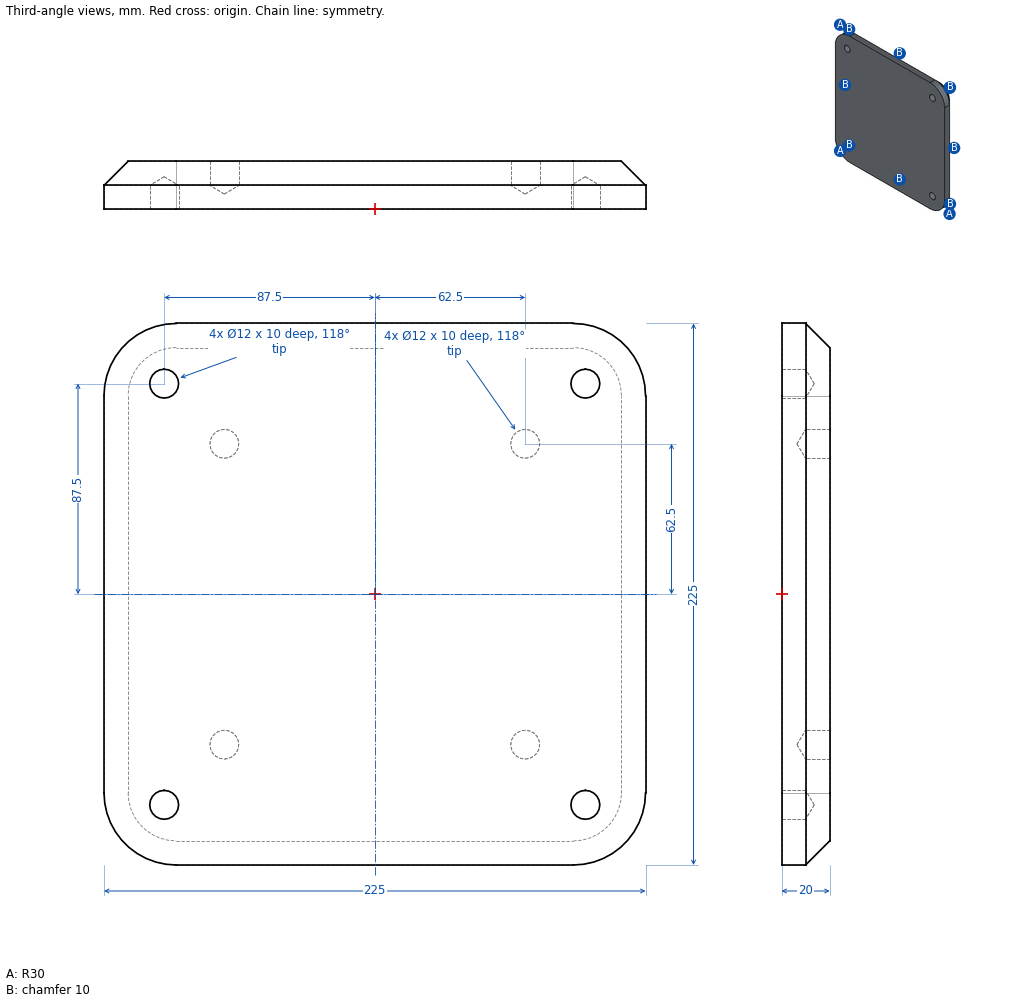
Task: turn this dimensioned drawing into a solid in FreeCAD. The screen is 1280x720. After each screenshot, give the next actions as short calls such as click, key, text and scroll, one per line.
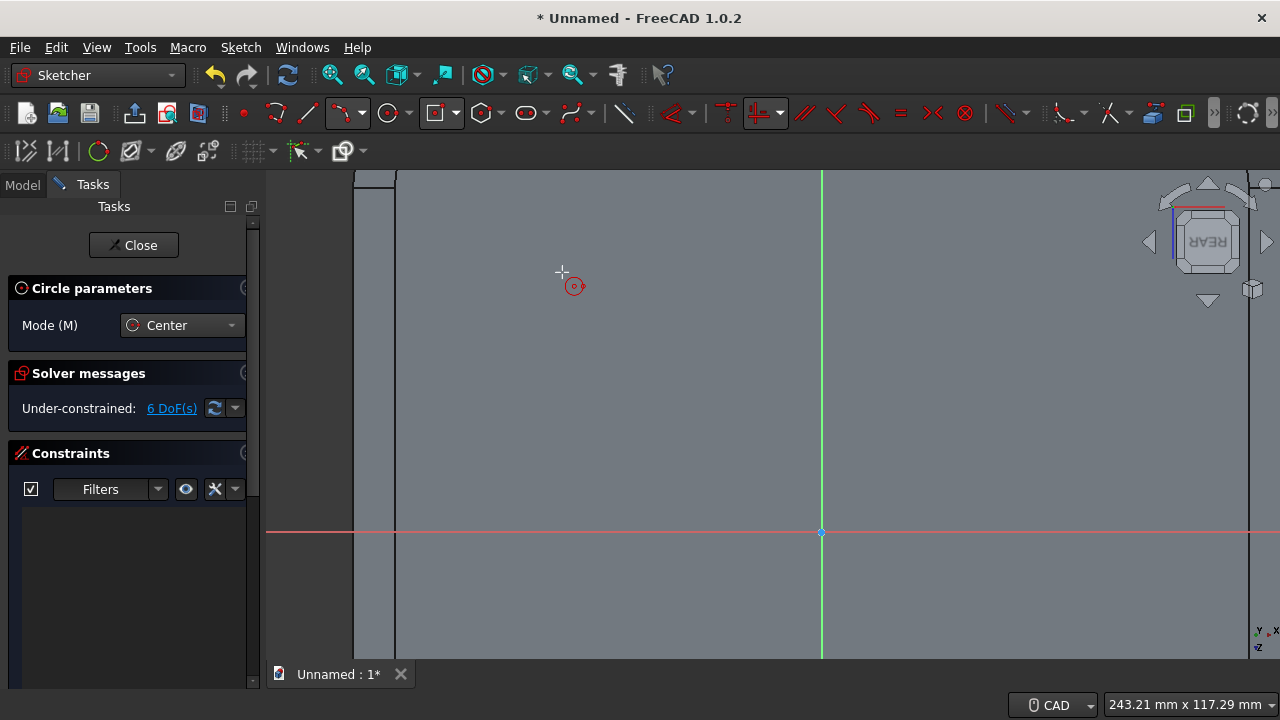
click(561, 272)
click(579, 254)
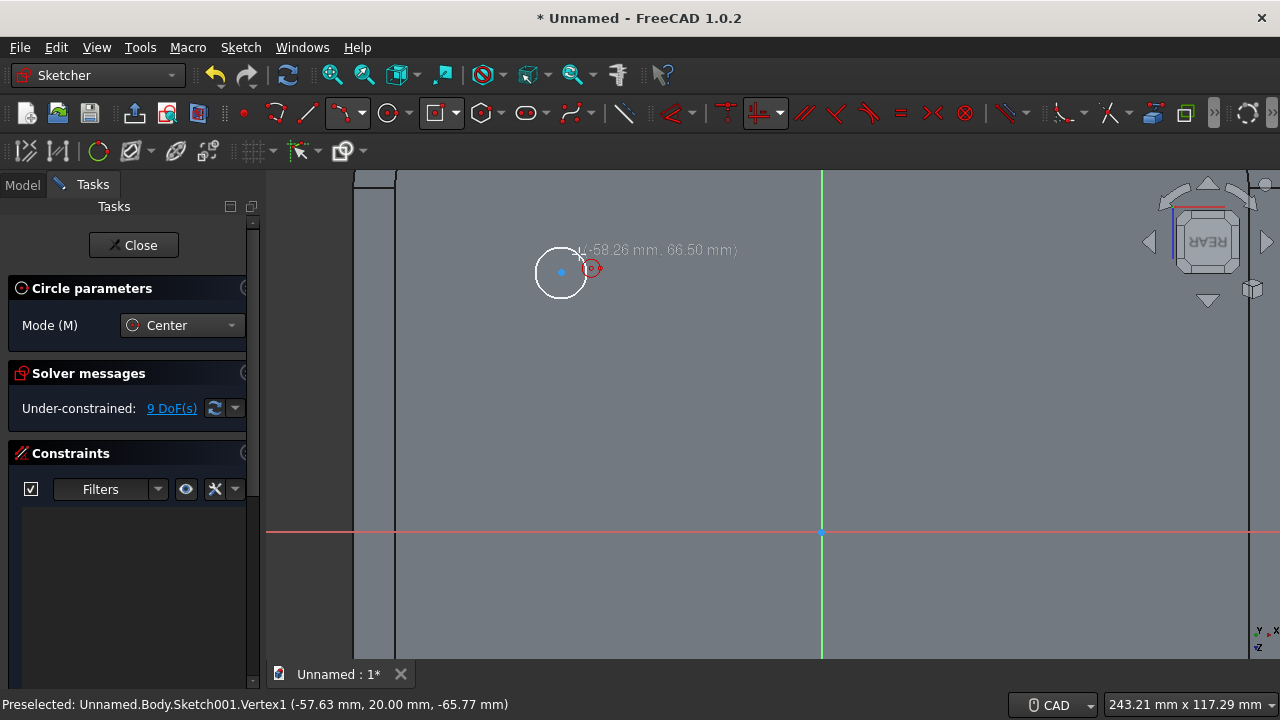
click(1082, 272)
click(1100, 254)
key(Escape)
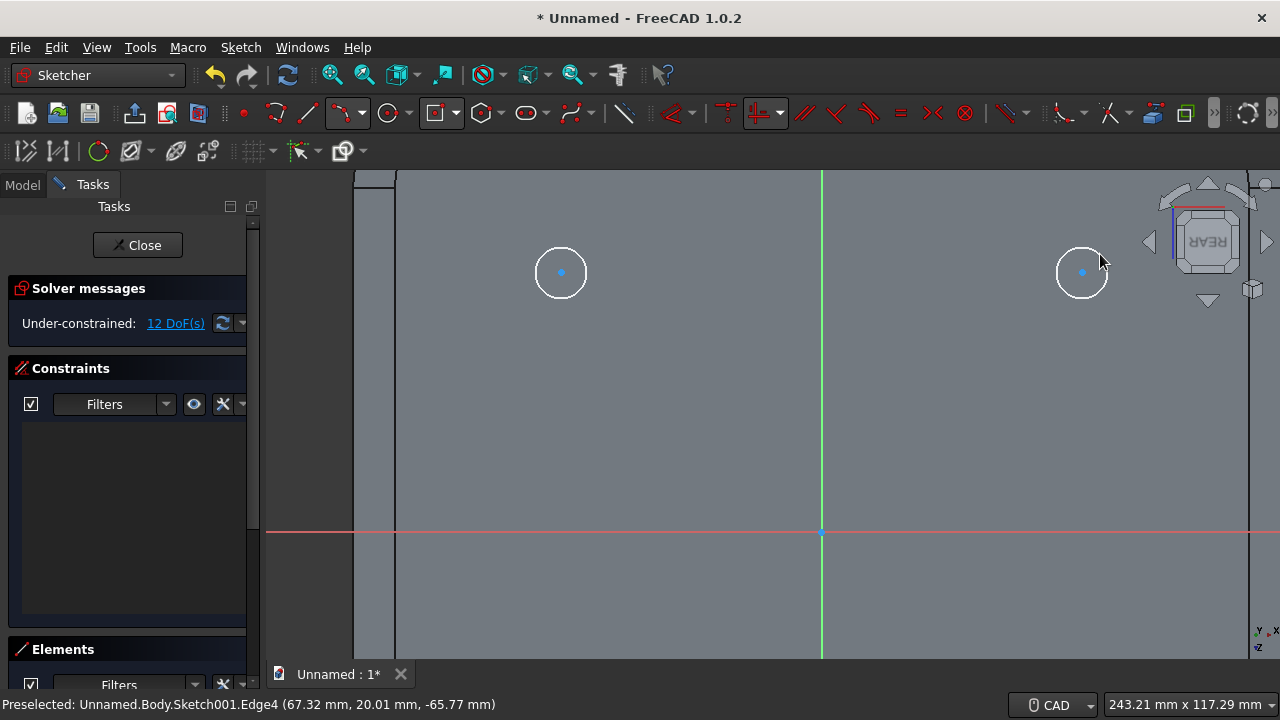
scroll(562, 271, down, 3)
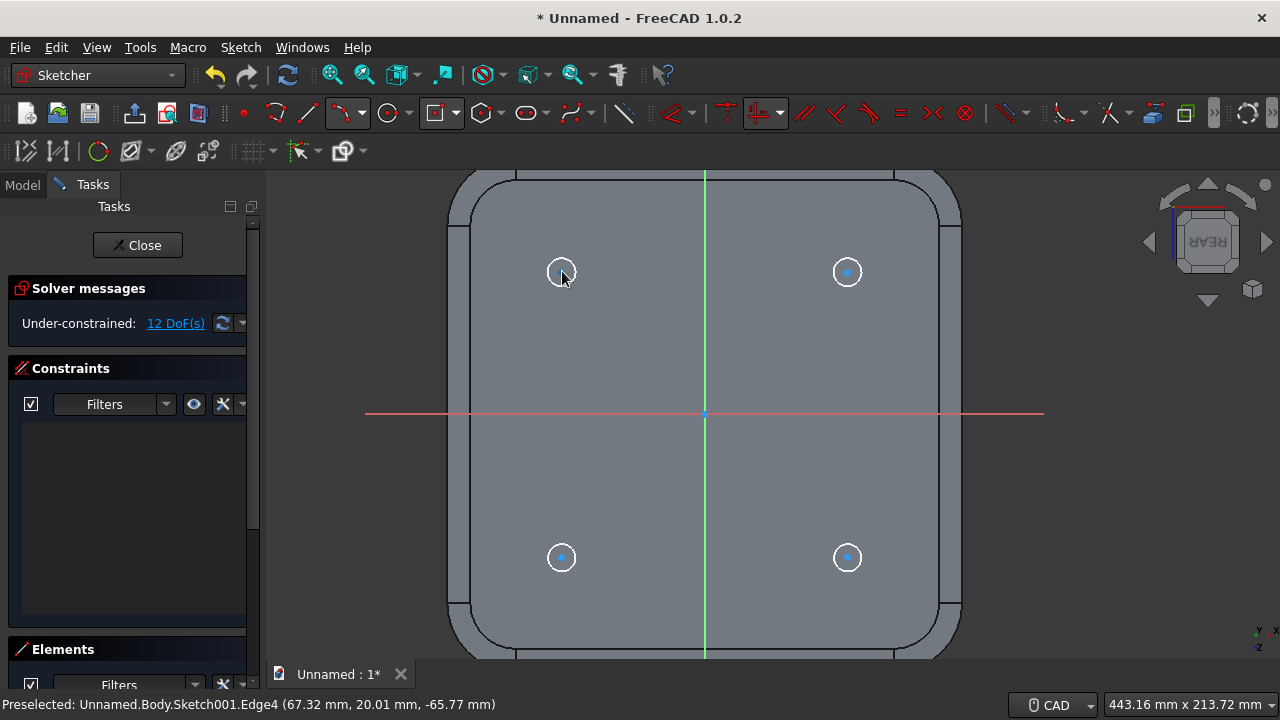
click(857, 548)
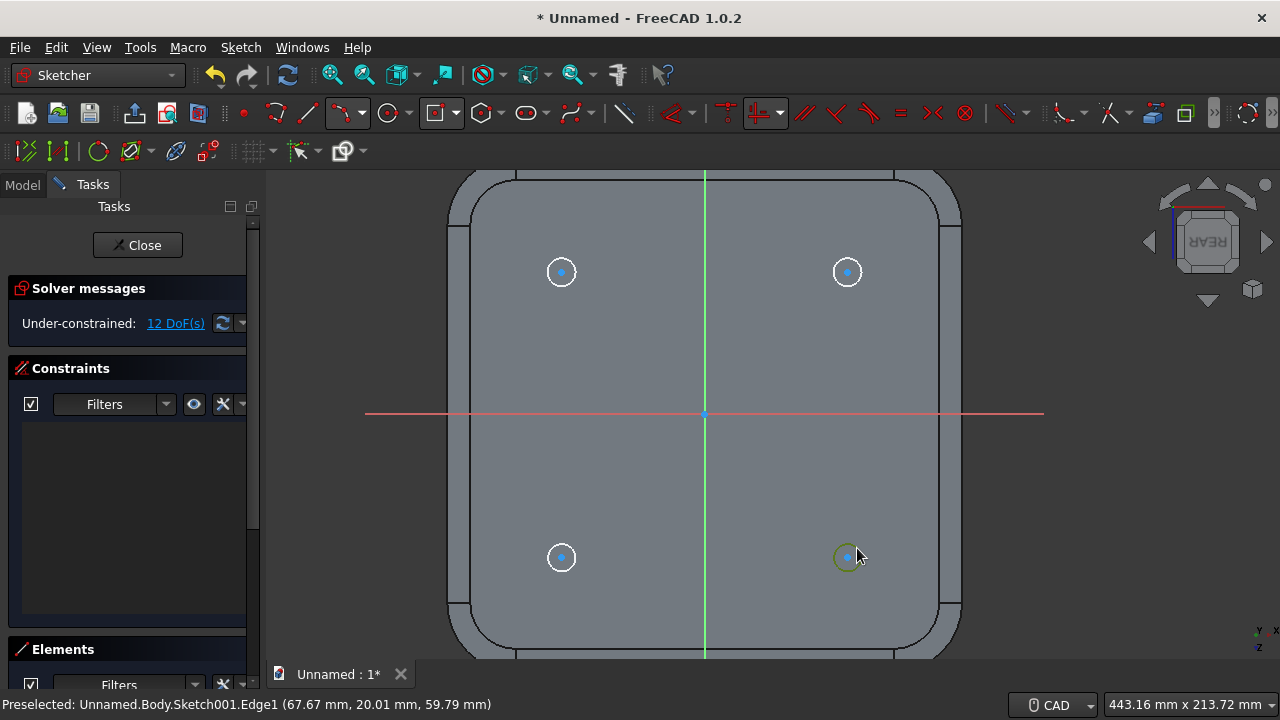
click(571, 548)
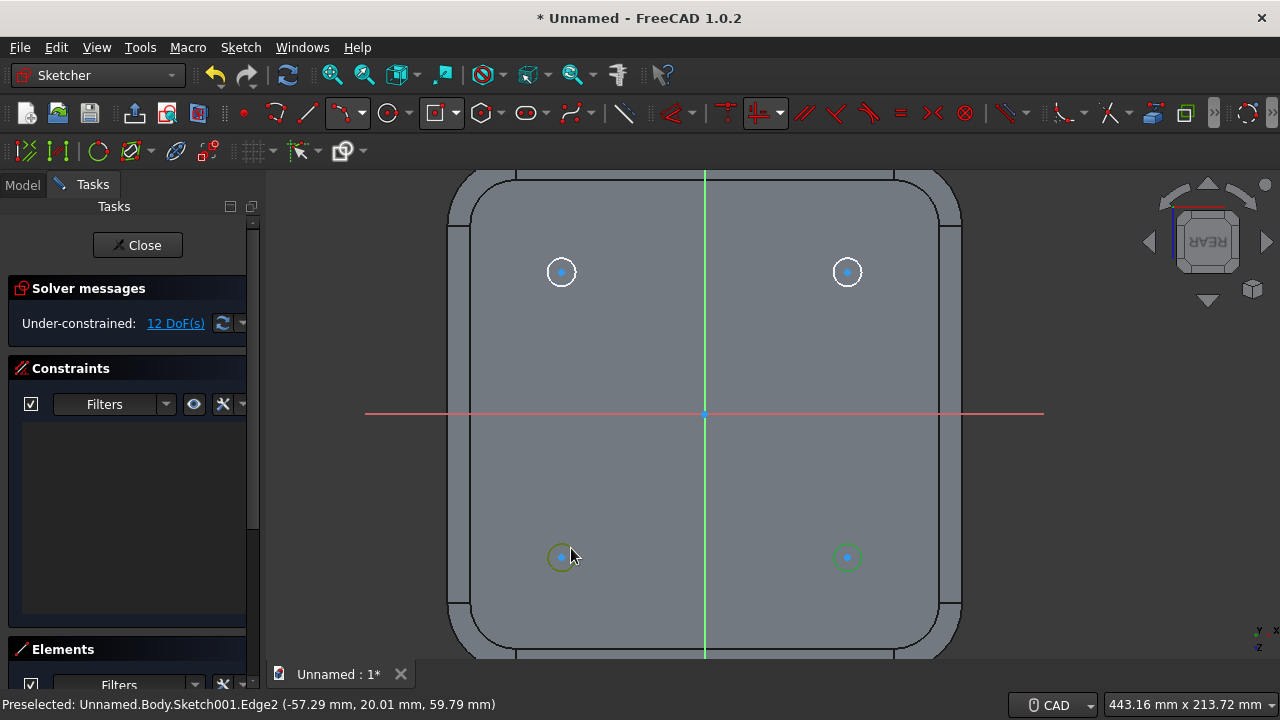
click(571, 262)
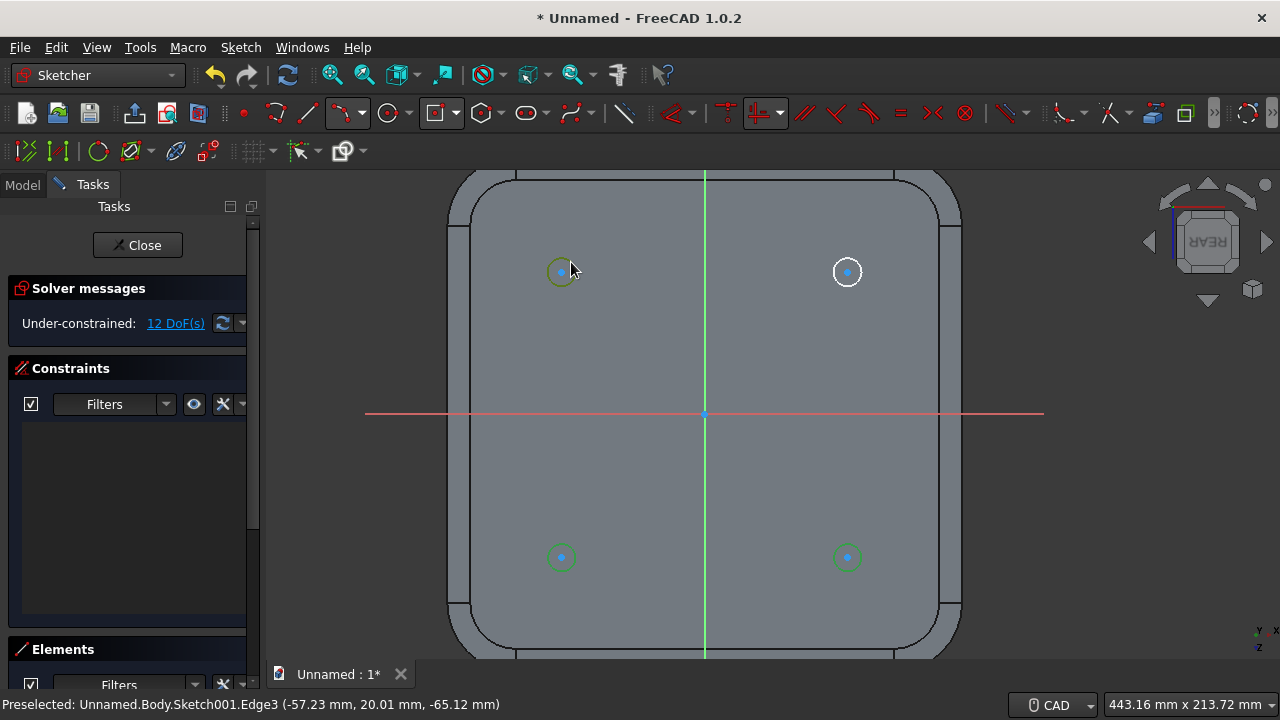
click(857, 262)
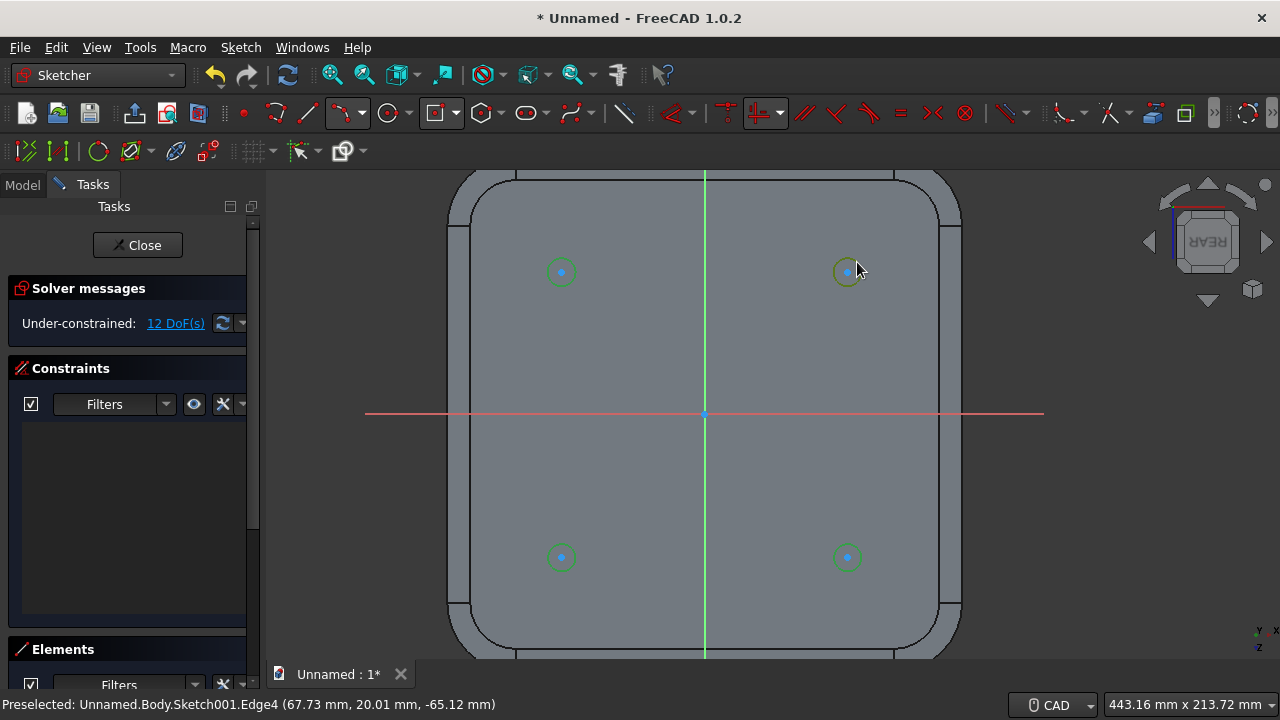
click(902, 114)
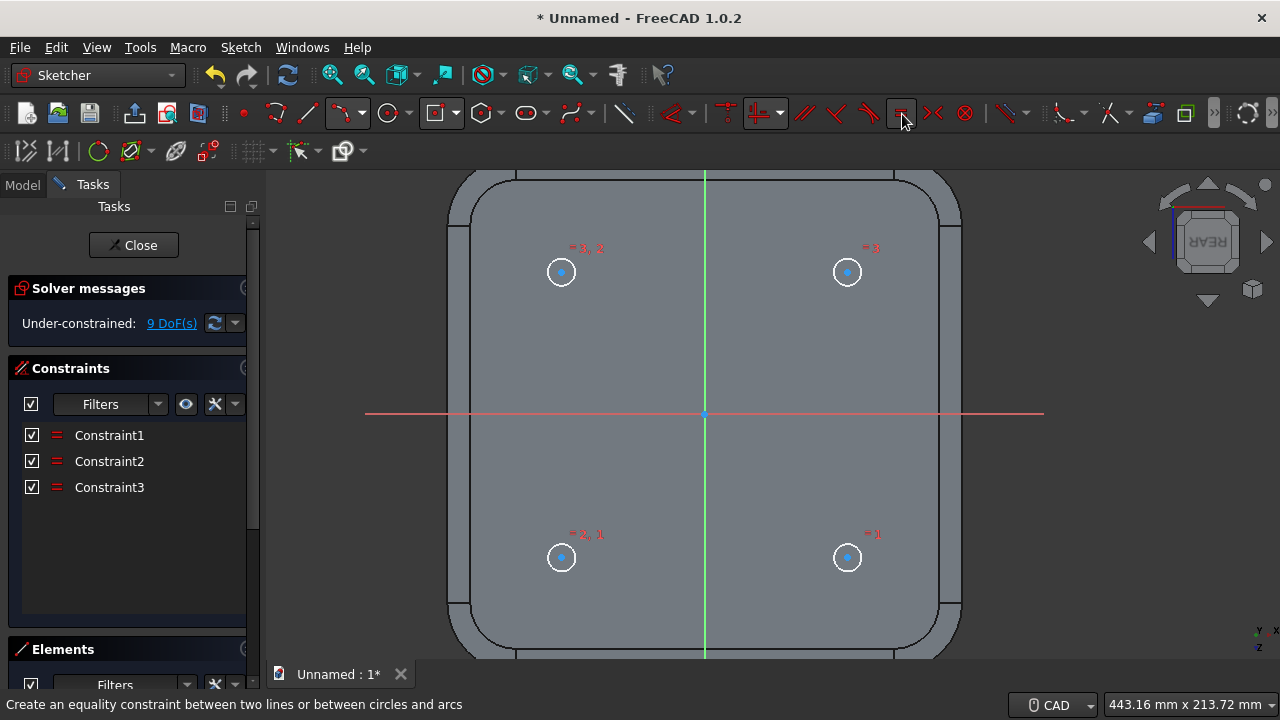
click(848, 558)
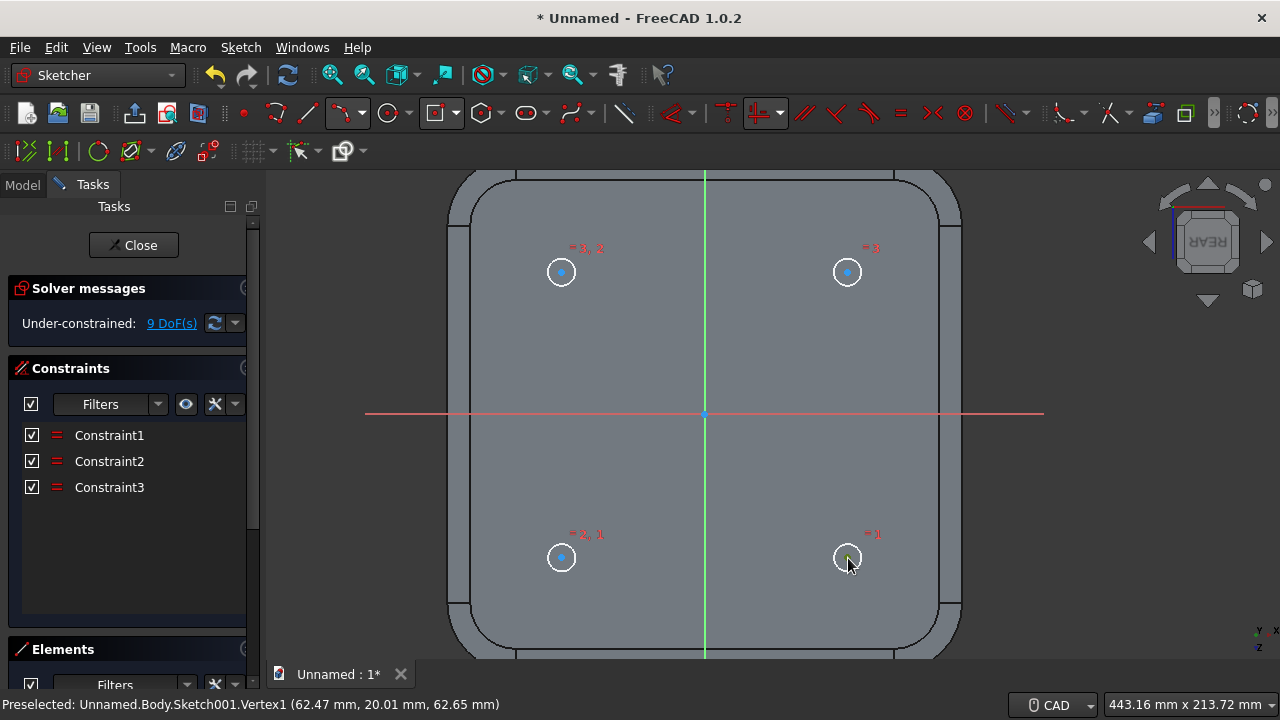
click(562, 558)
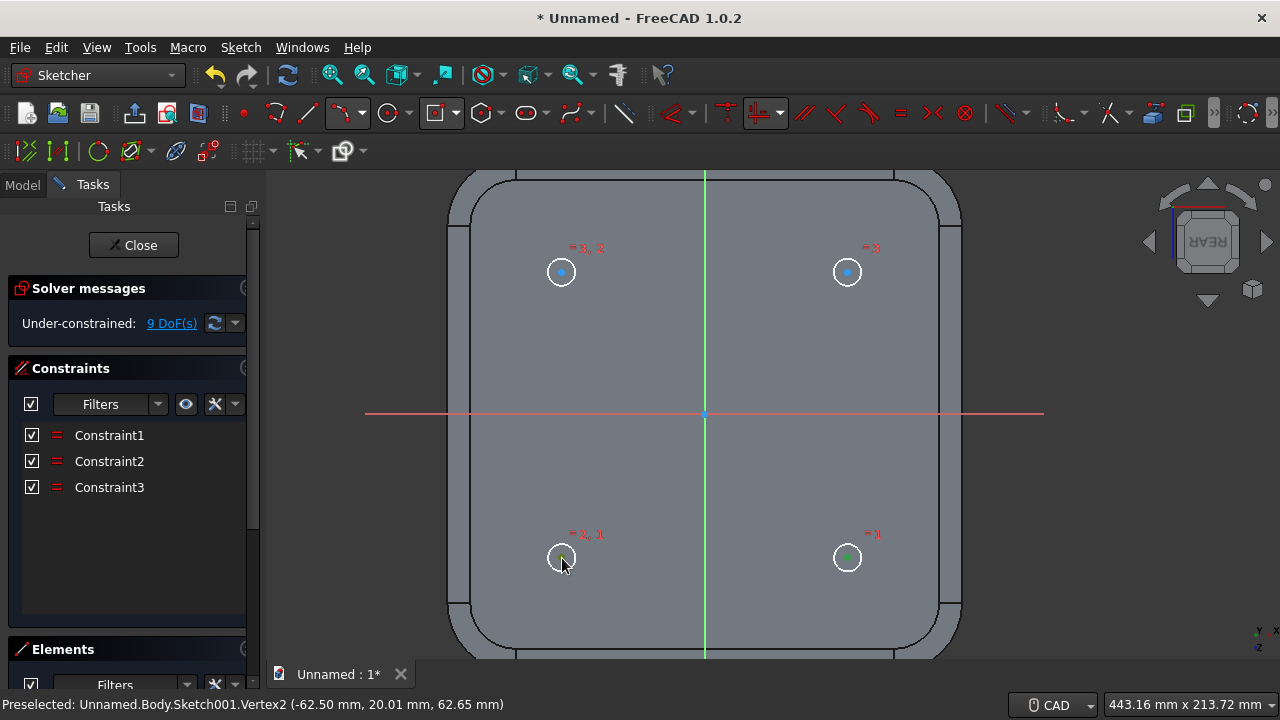
click(705, 600)